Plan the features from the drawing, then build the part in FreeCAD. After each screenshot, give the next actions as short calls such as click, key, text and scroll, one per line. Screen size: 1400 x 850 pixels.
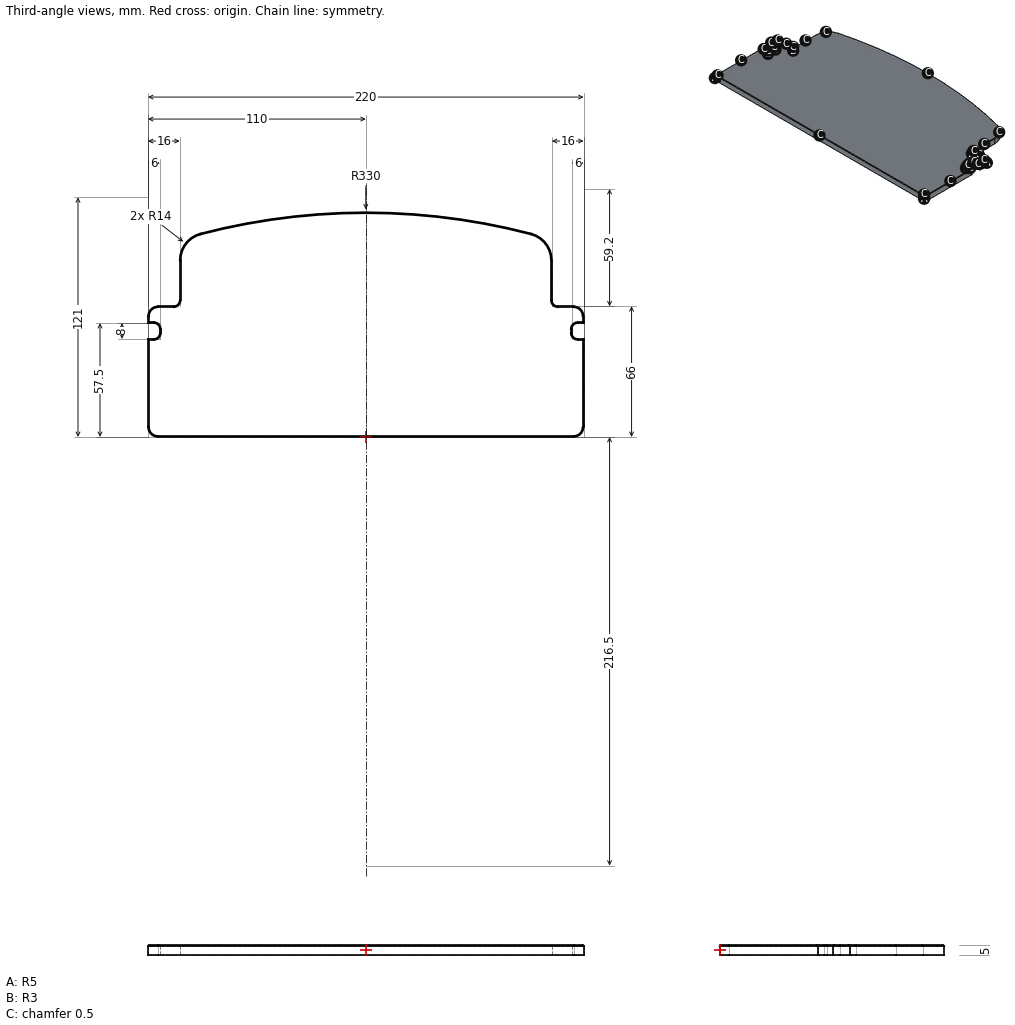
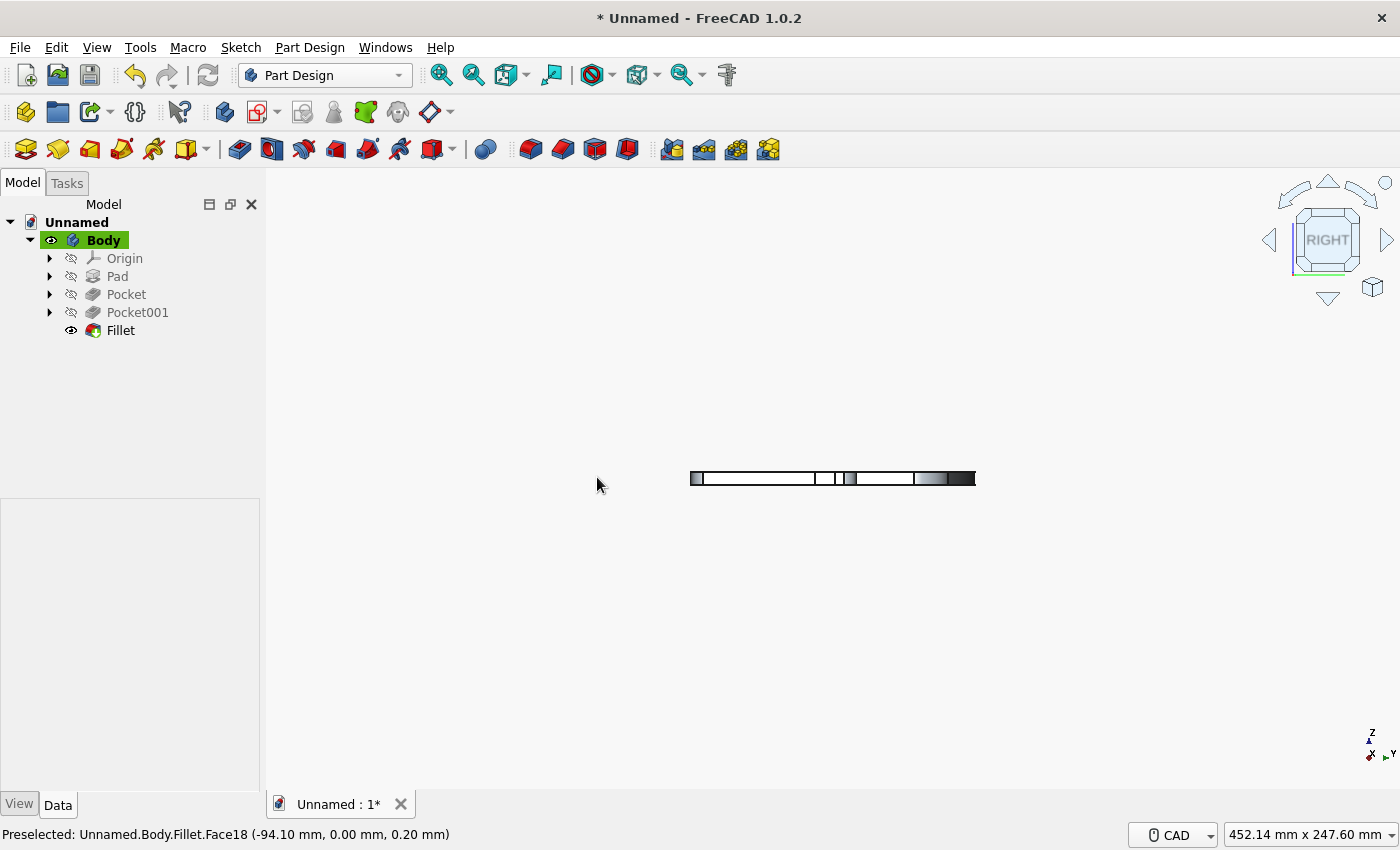
click(442, 76)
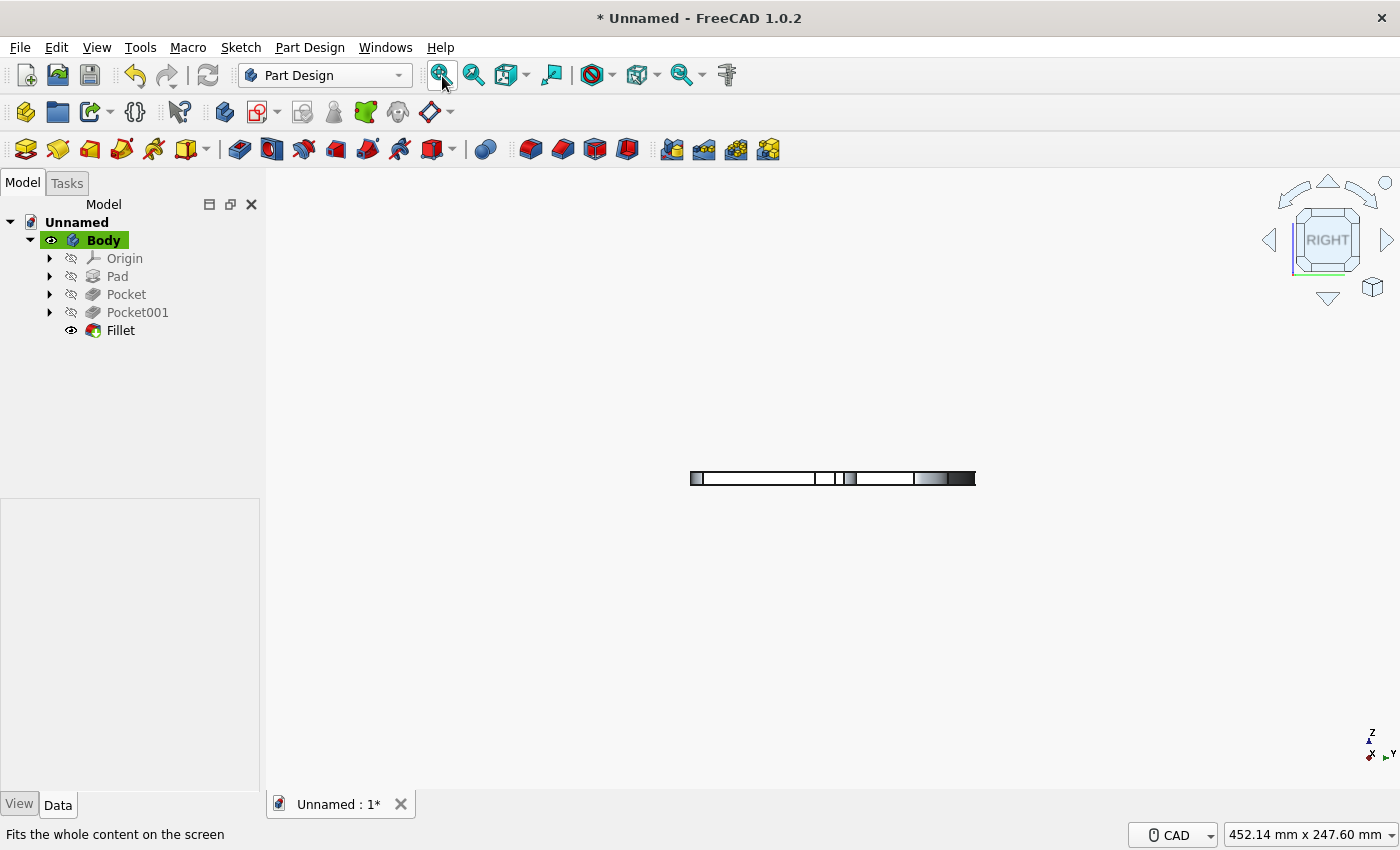
scroll(856, 477, up, 6)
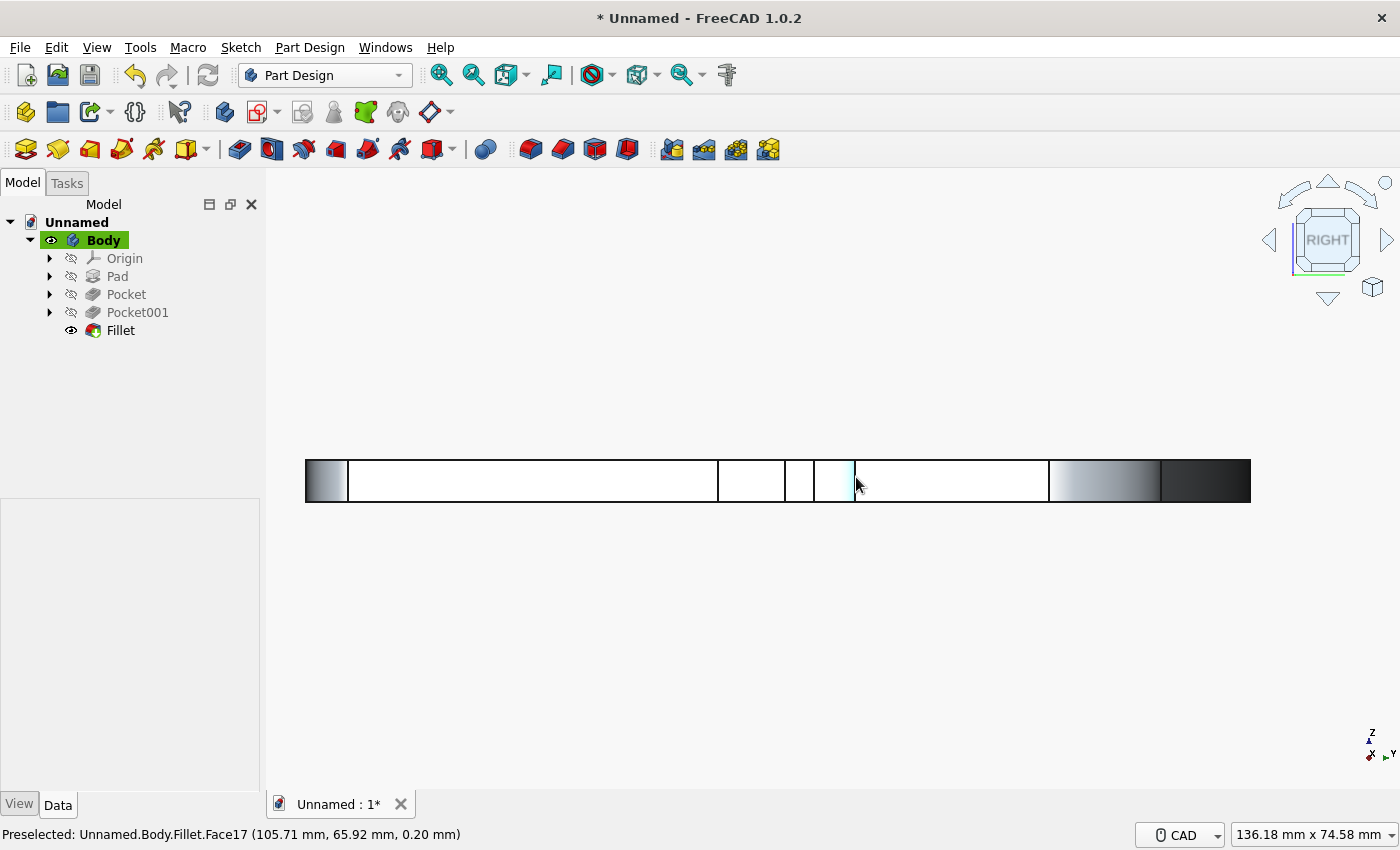
key(v)
key(f)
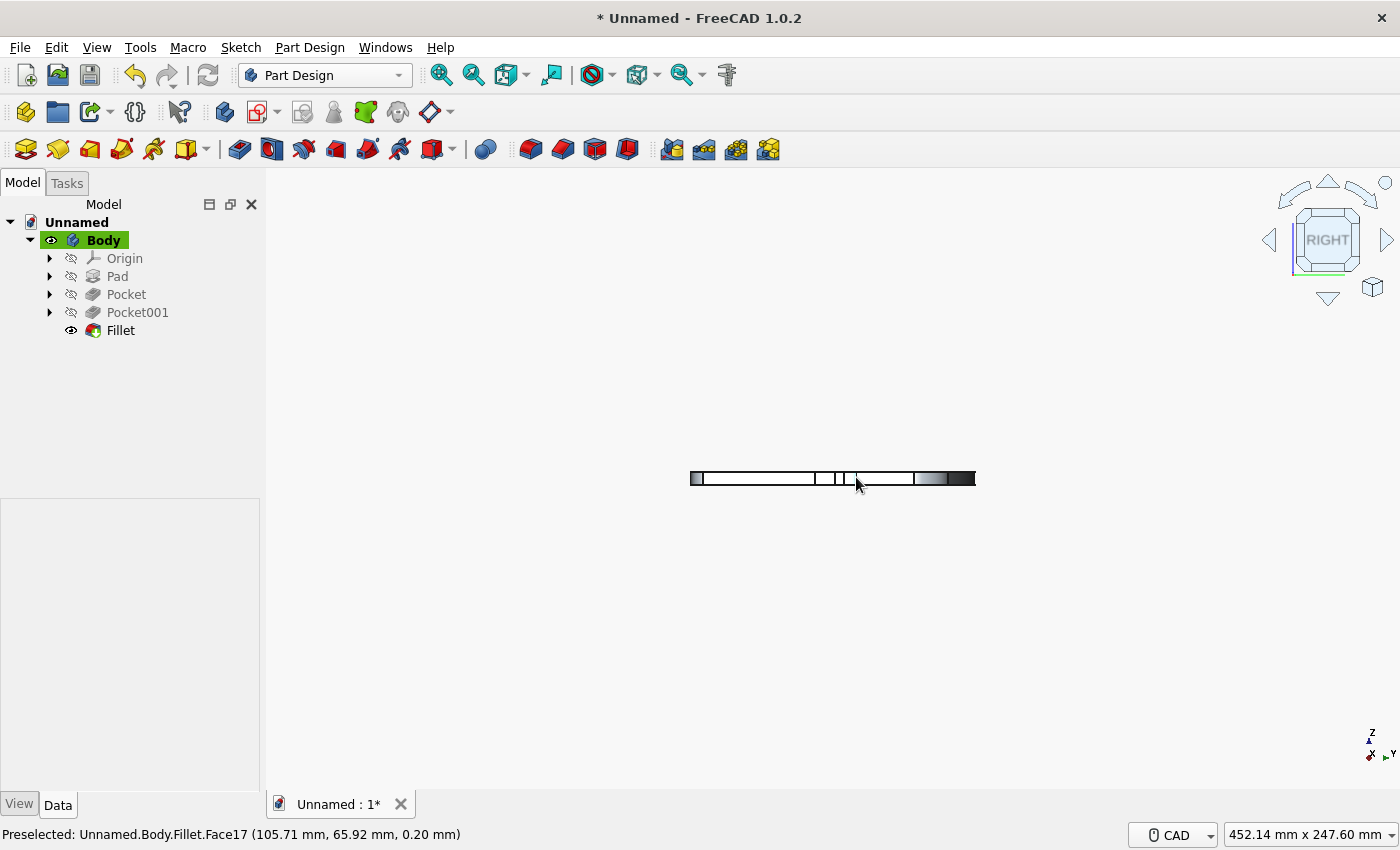
key(5)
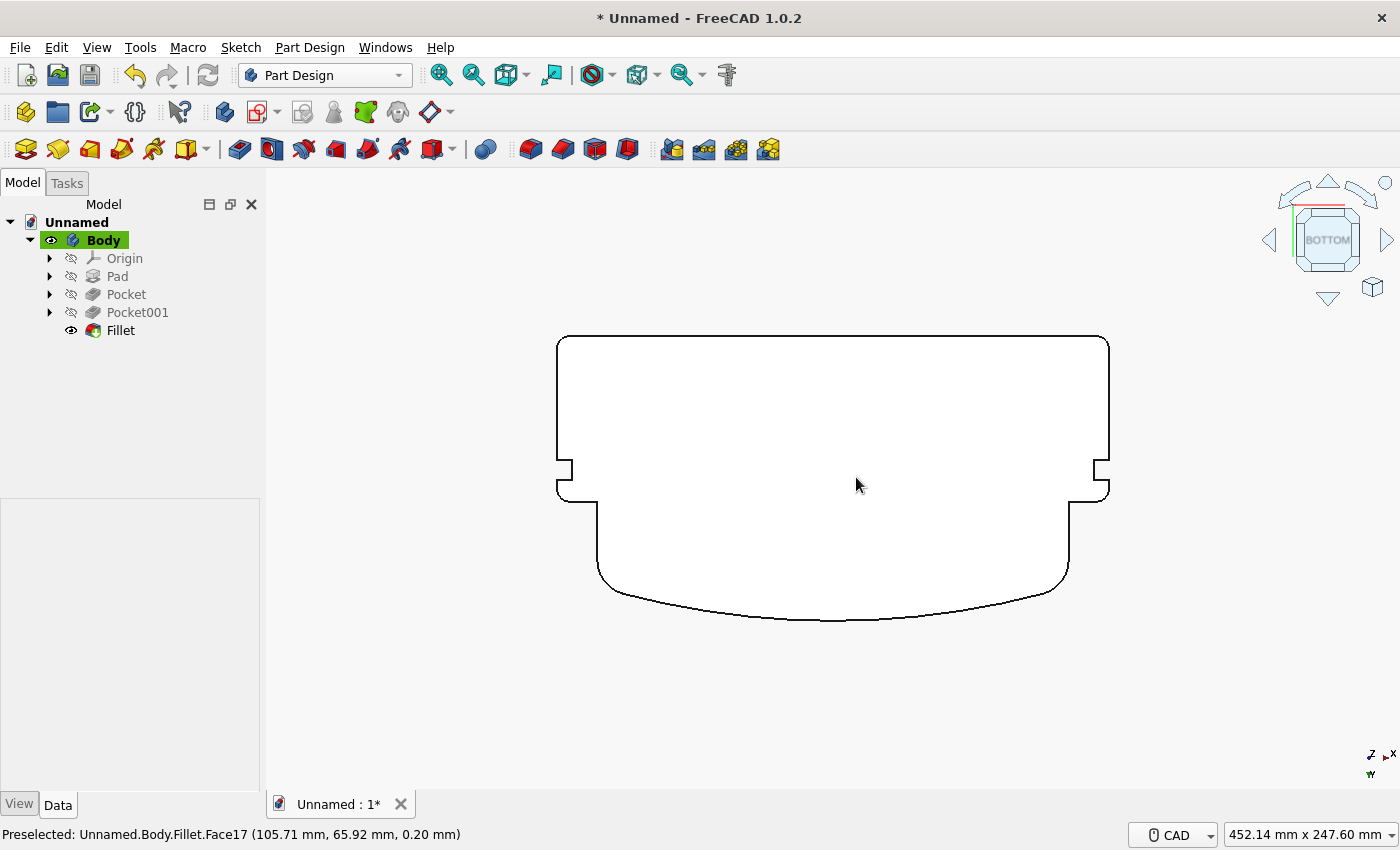
scroll(597, 501, up, 6)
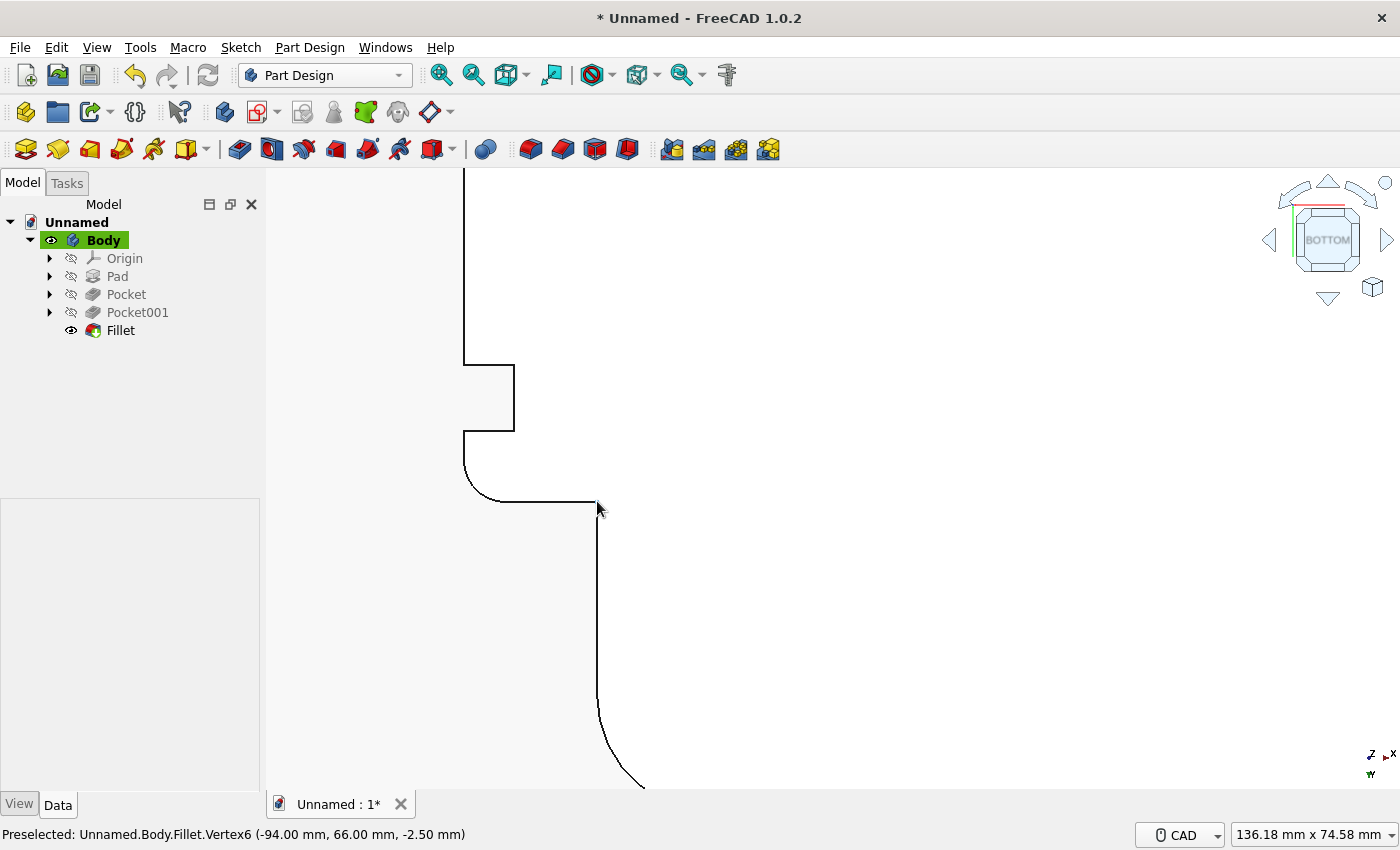
key(v)
key(f)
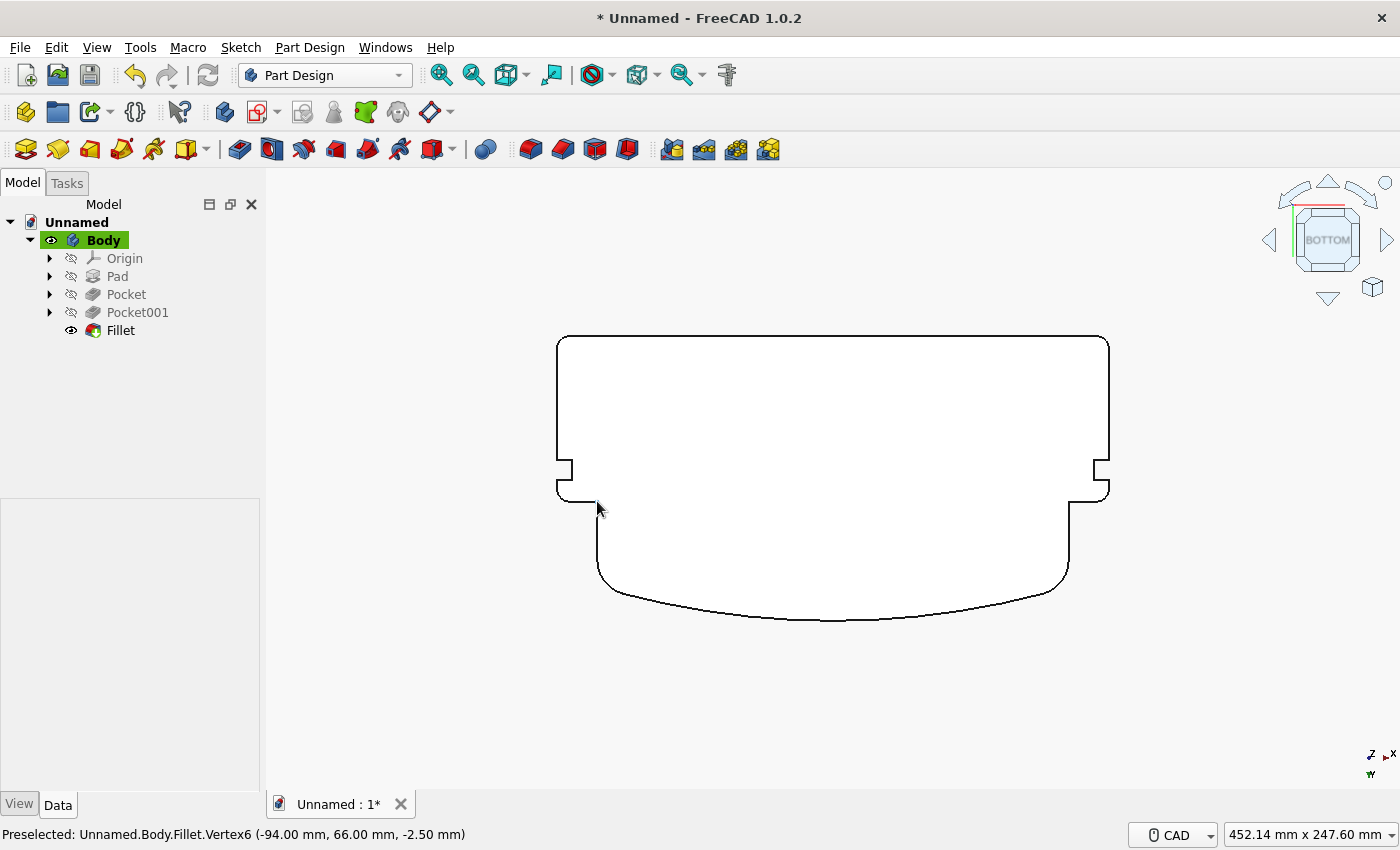
key(4)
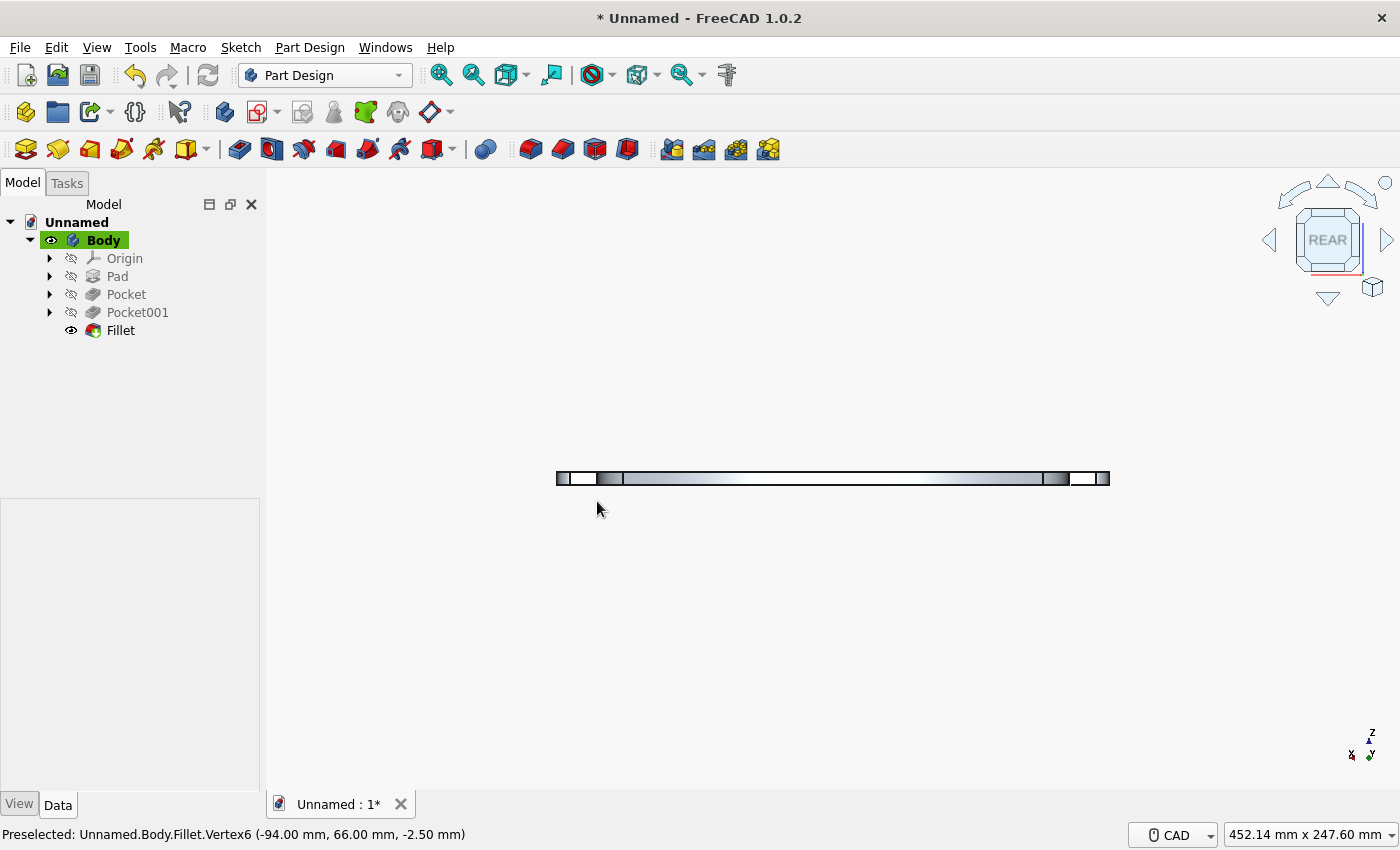
scroll(1069, 477, up, 6)